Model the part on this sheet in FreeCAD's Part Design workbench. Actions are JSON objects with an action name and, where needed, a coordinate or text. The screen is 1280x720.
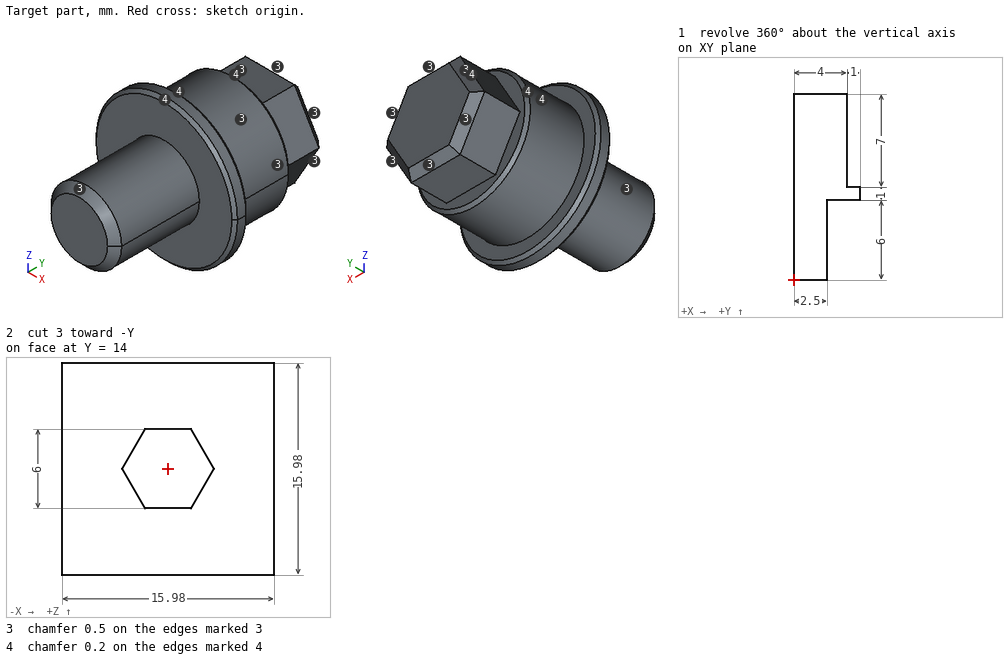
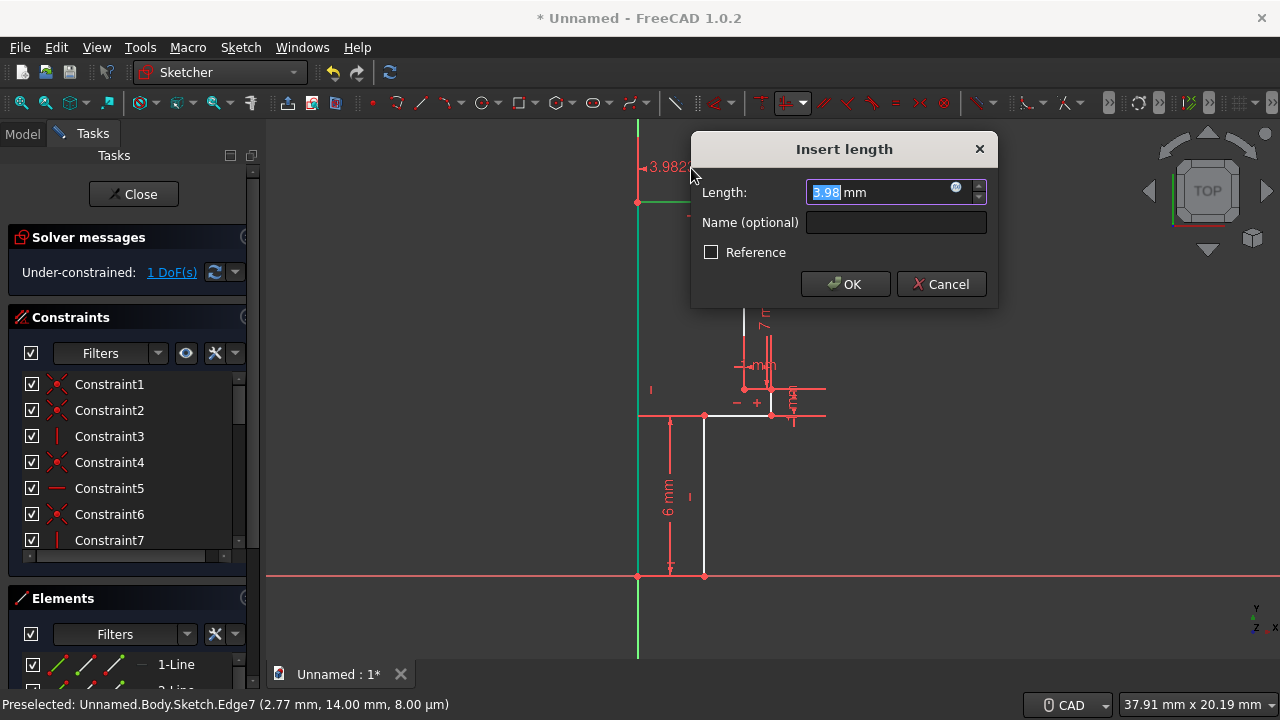
{"action": "type", "text": "4"}
{"action": "key", "text": "Return"}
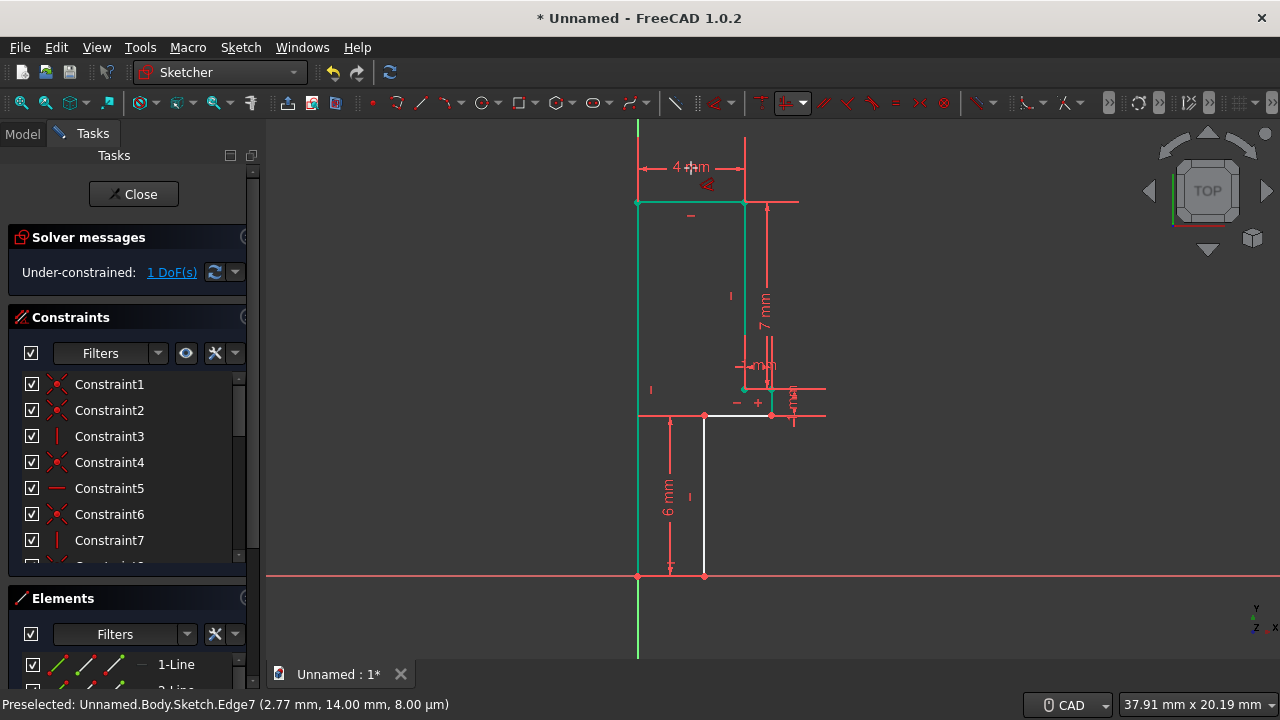
{"action": "left_click", "coordinate": [658, 576]}
{"action": "left_click", "coordinate": [671, 610]}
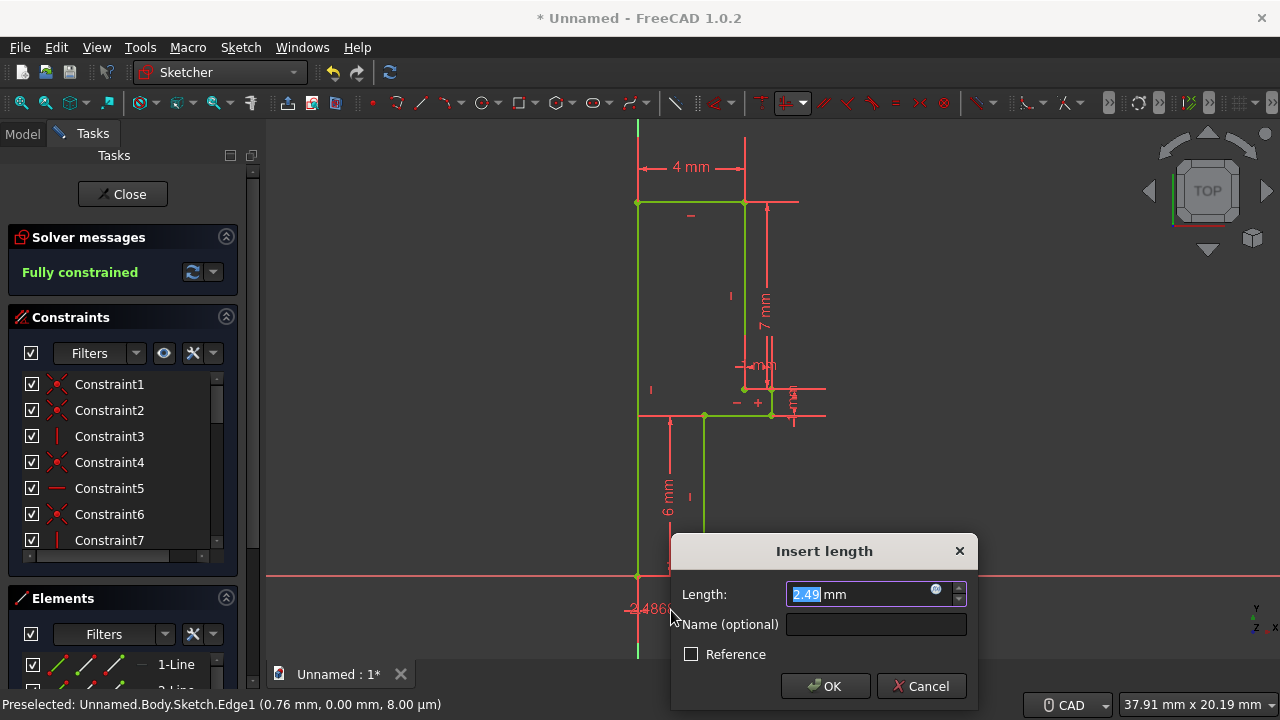
{"action": "type", "text": "2.5"}
{"action": "key", "text": "Return"}
{"action": "key", "text": "Escape"}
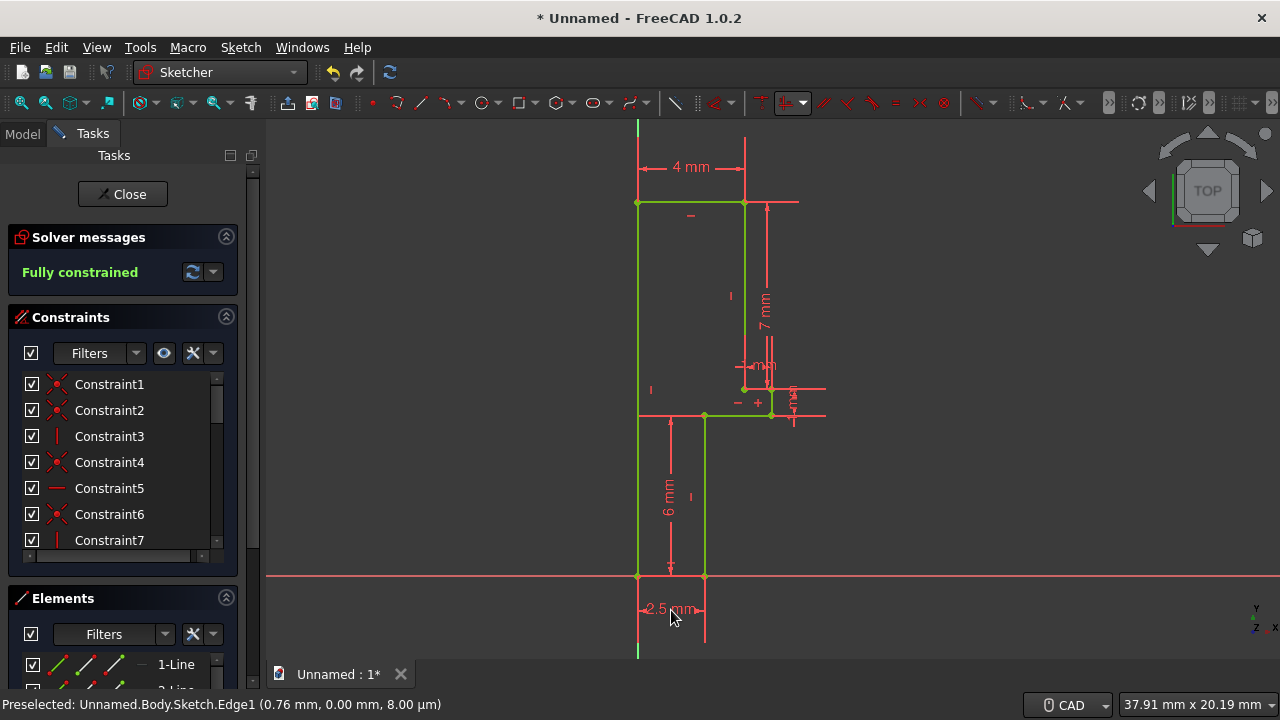
{"action": "left_click", "coordinate": [123, 194]}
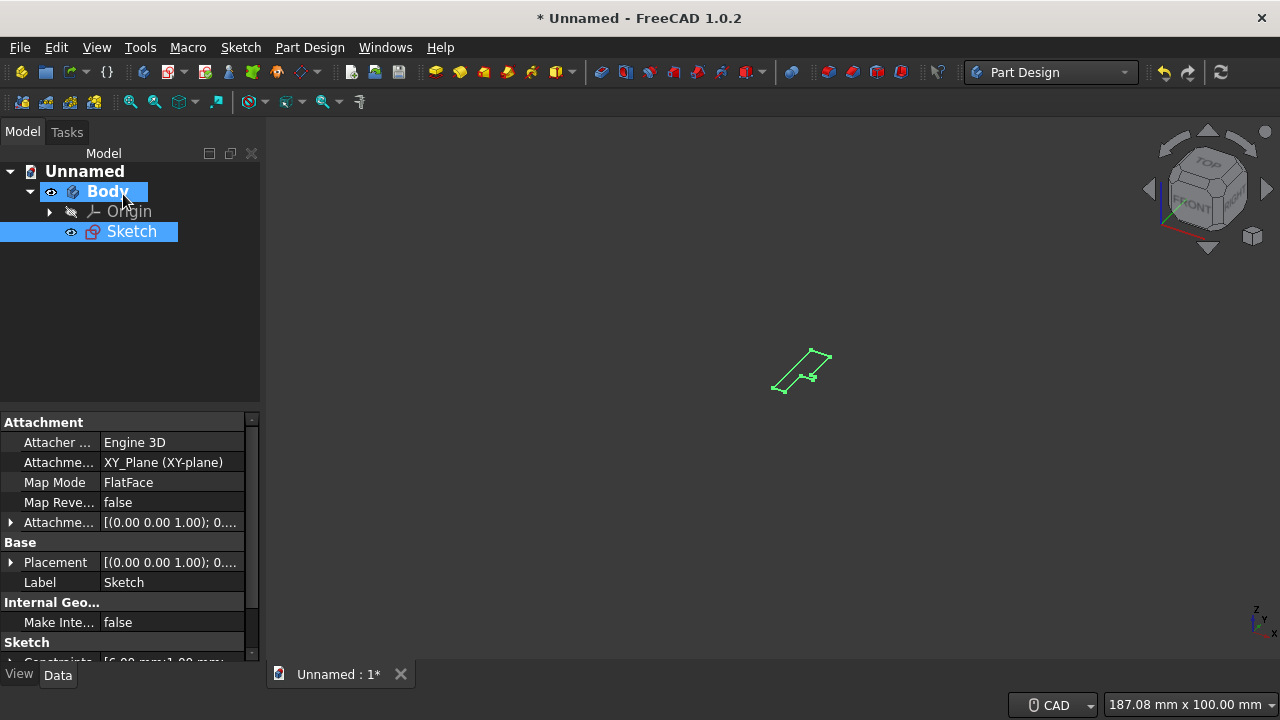
{"action": "left_click", "coordinate": [460, 72]}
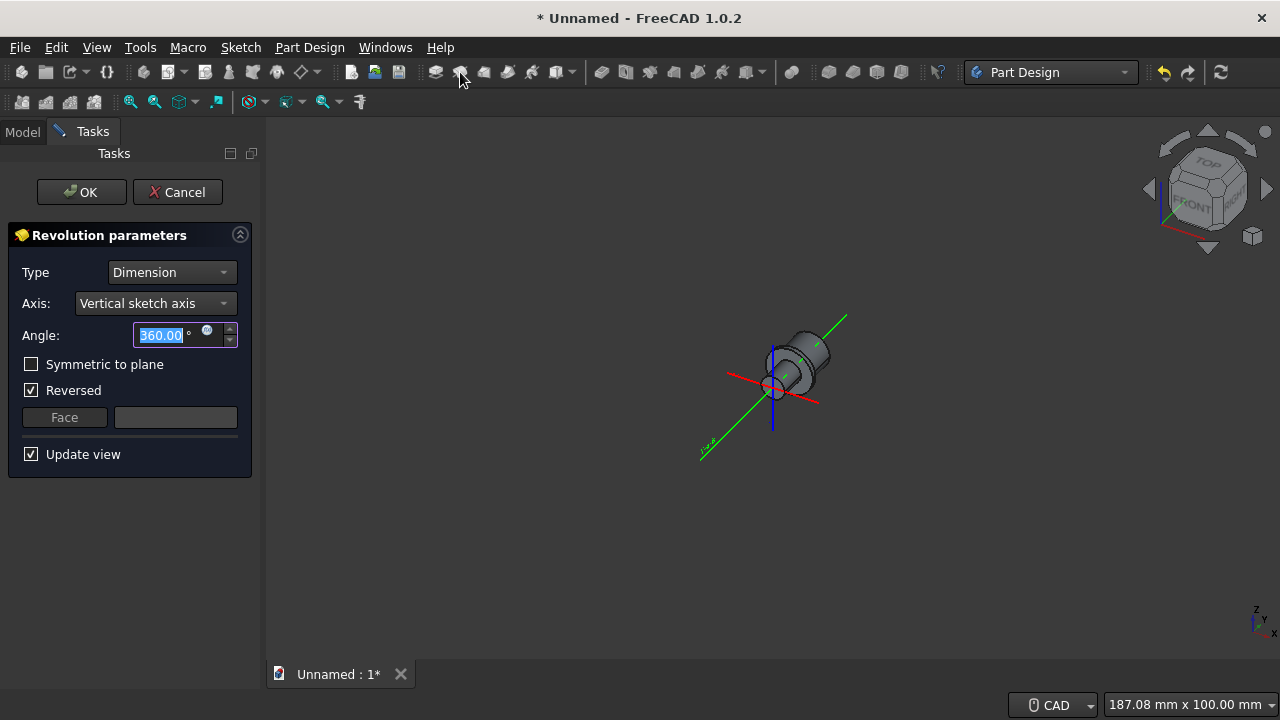
{"action": "left_click", "coordinate": [82, 192]}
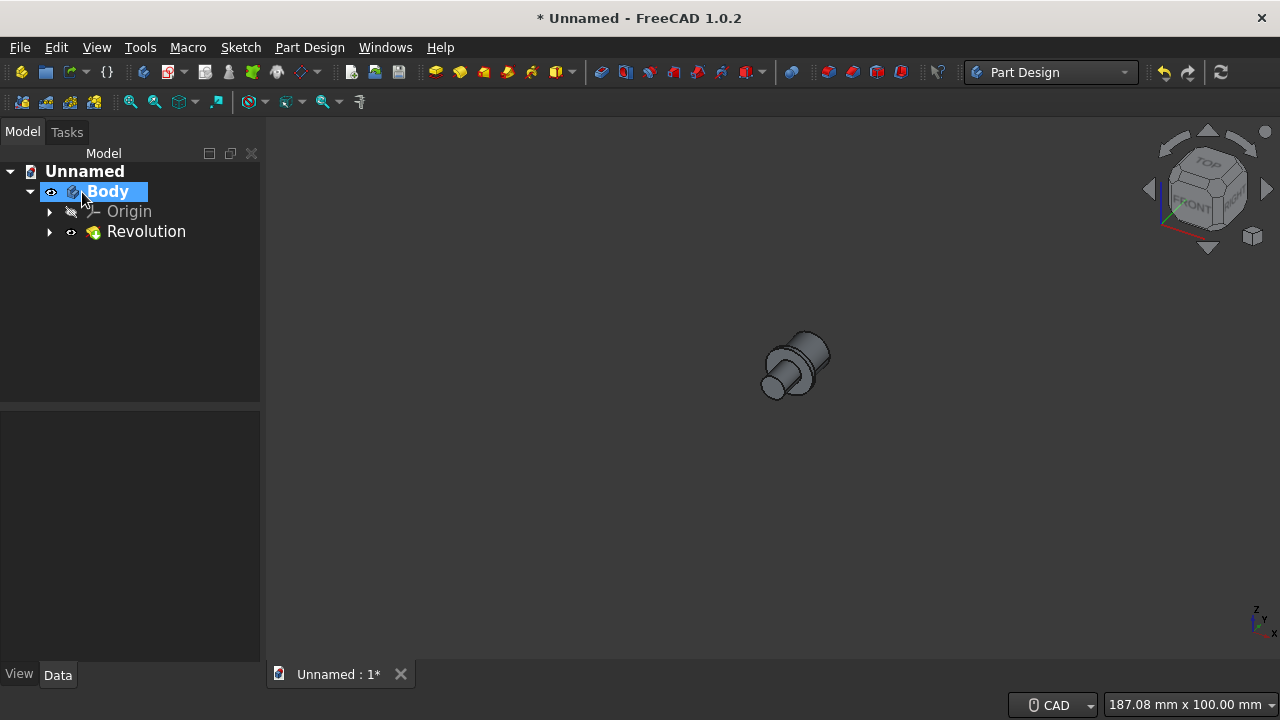
{"action": "left_click", "coordinate": [132, 102]}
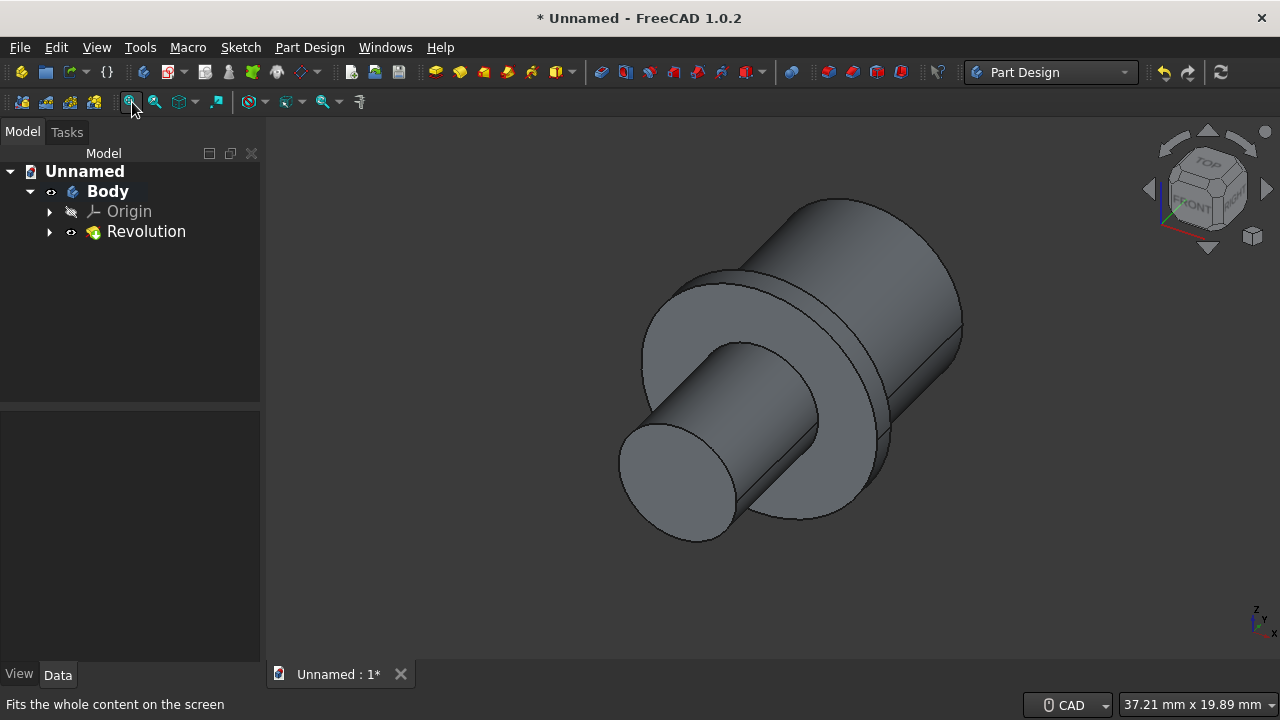
{"action": "key", "text": "4"}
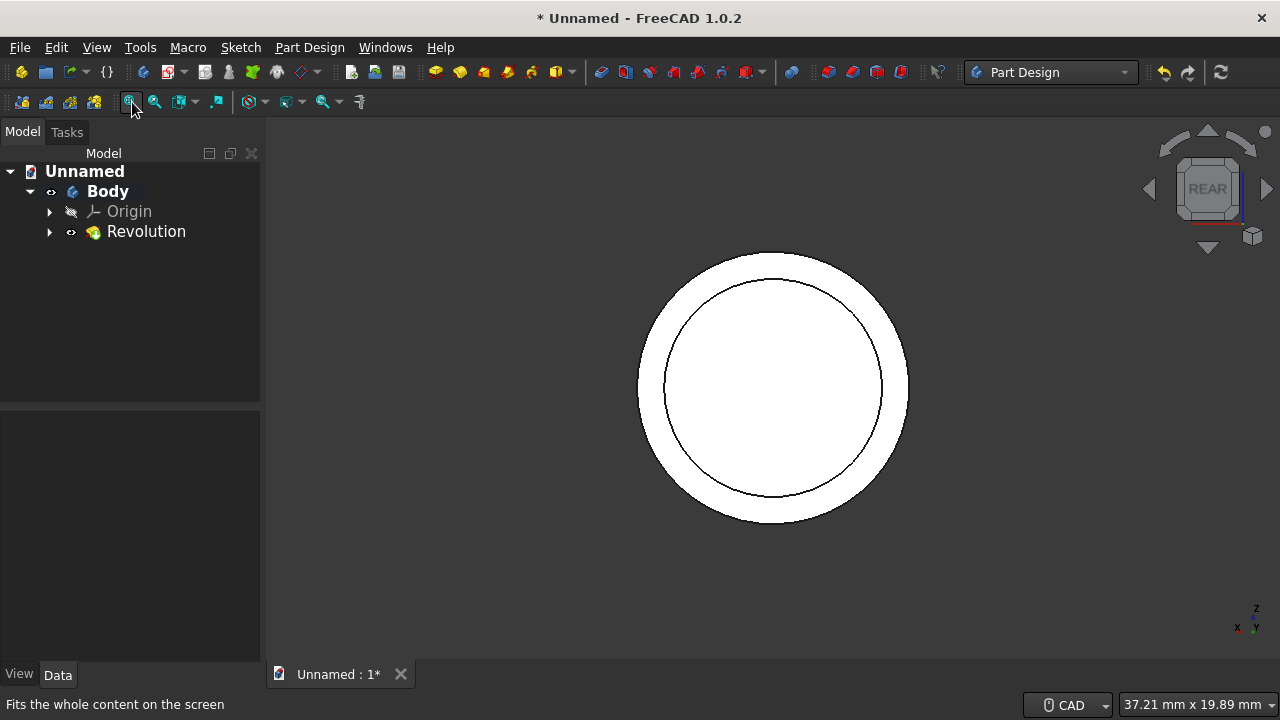
{"action": "left_click", "coordinate": [773, 387]}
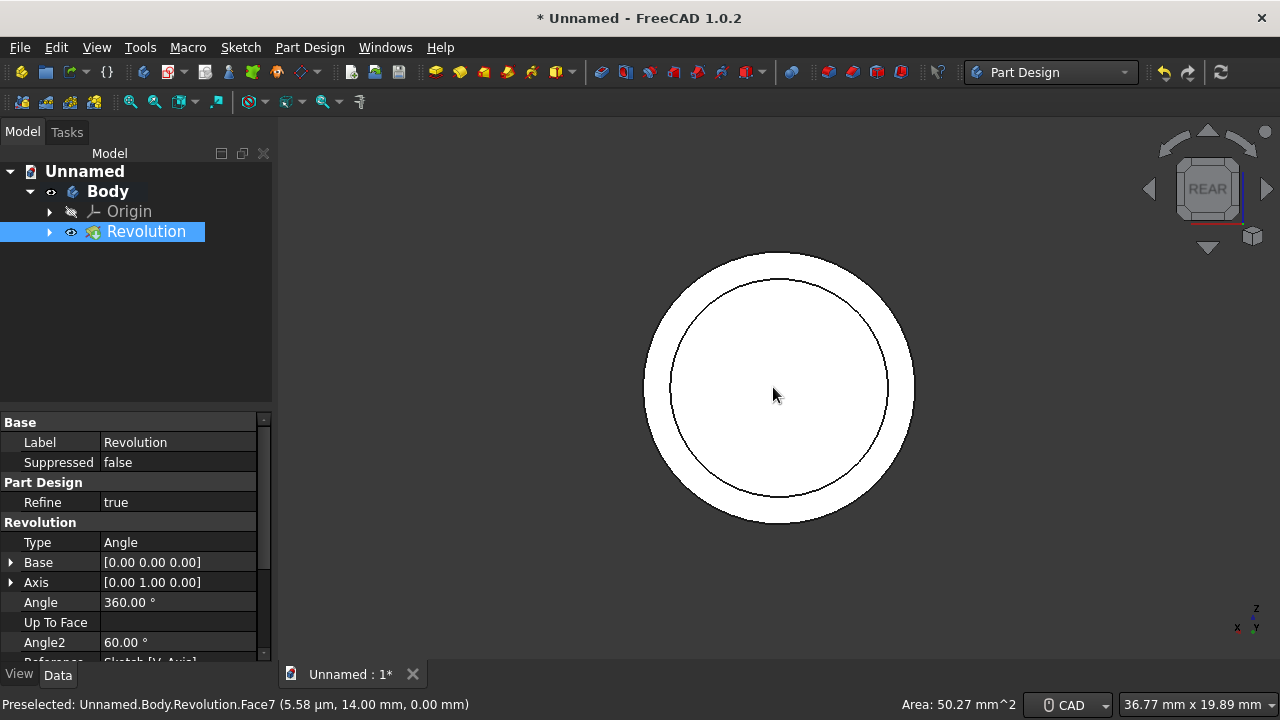
{"action": "left_click", "coordinate": [168, 72]}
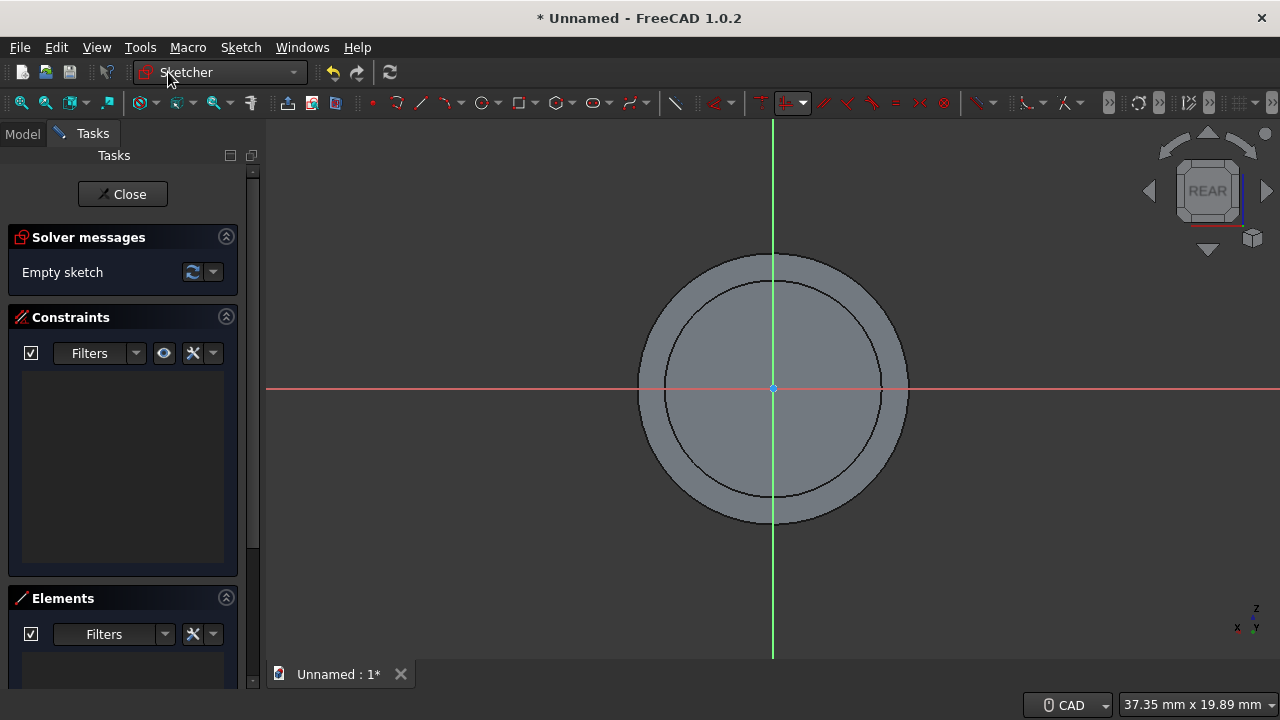
{"action": "key", "text": "g v"}